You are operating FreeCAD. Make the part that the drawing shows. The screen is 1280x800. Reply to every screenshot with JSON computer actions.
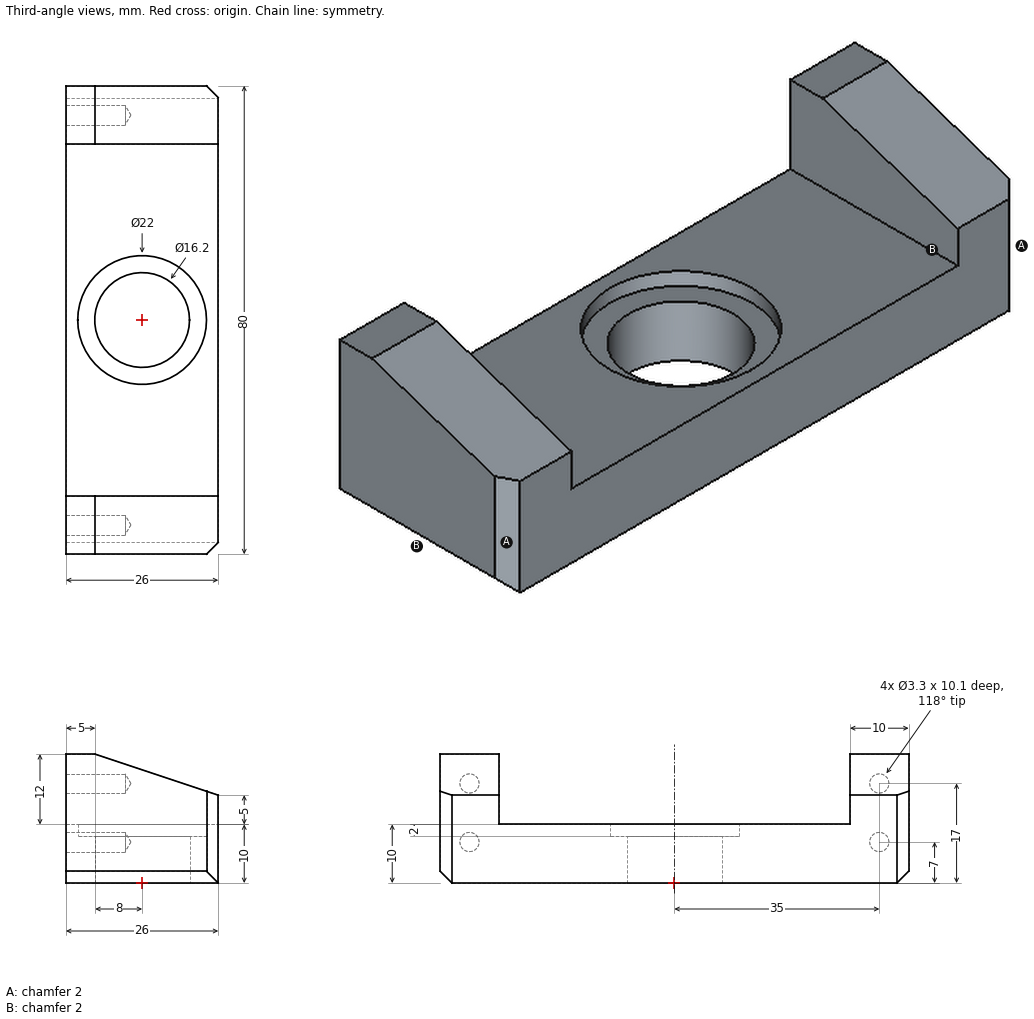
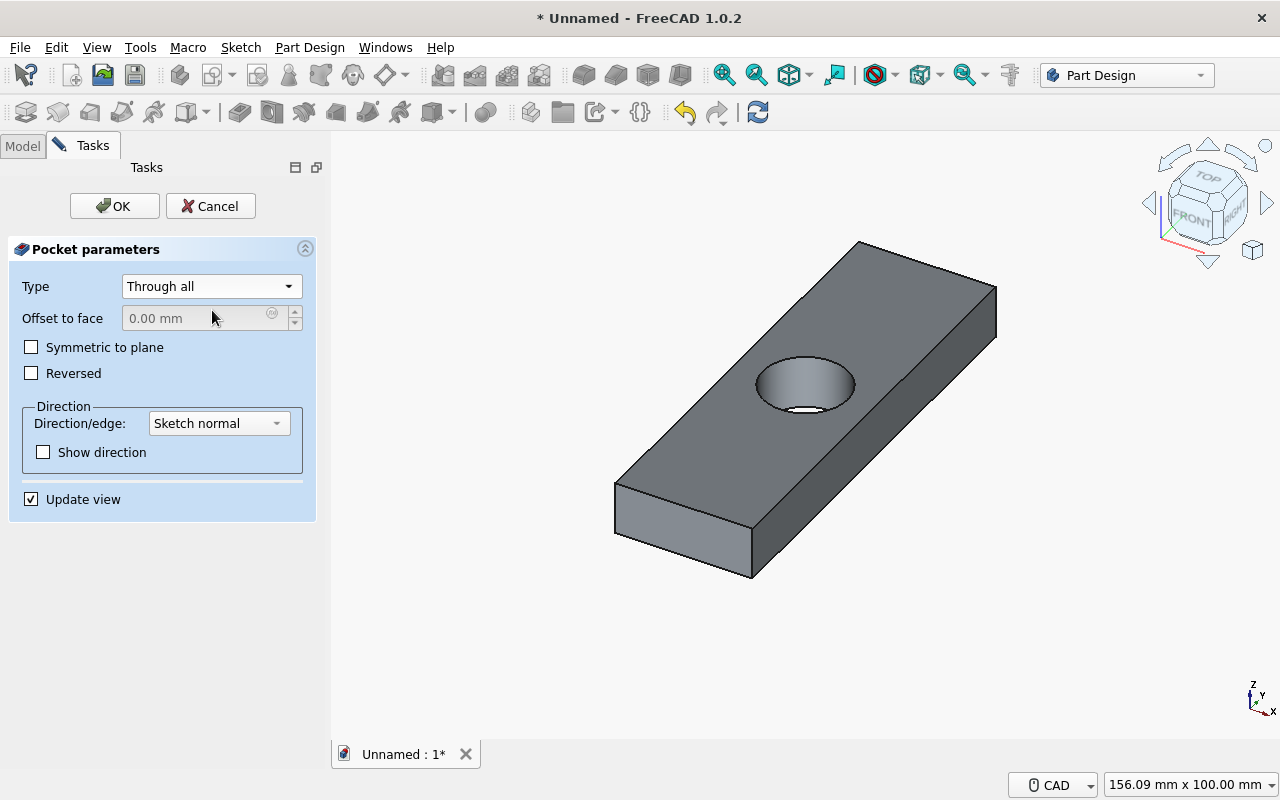
{"action": "left_click", "coordinate": [115, 206]}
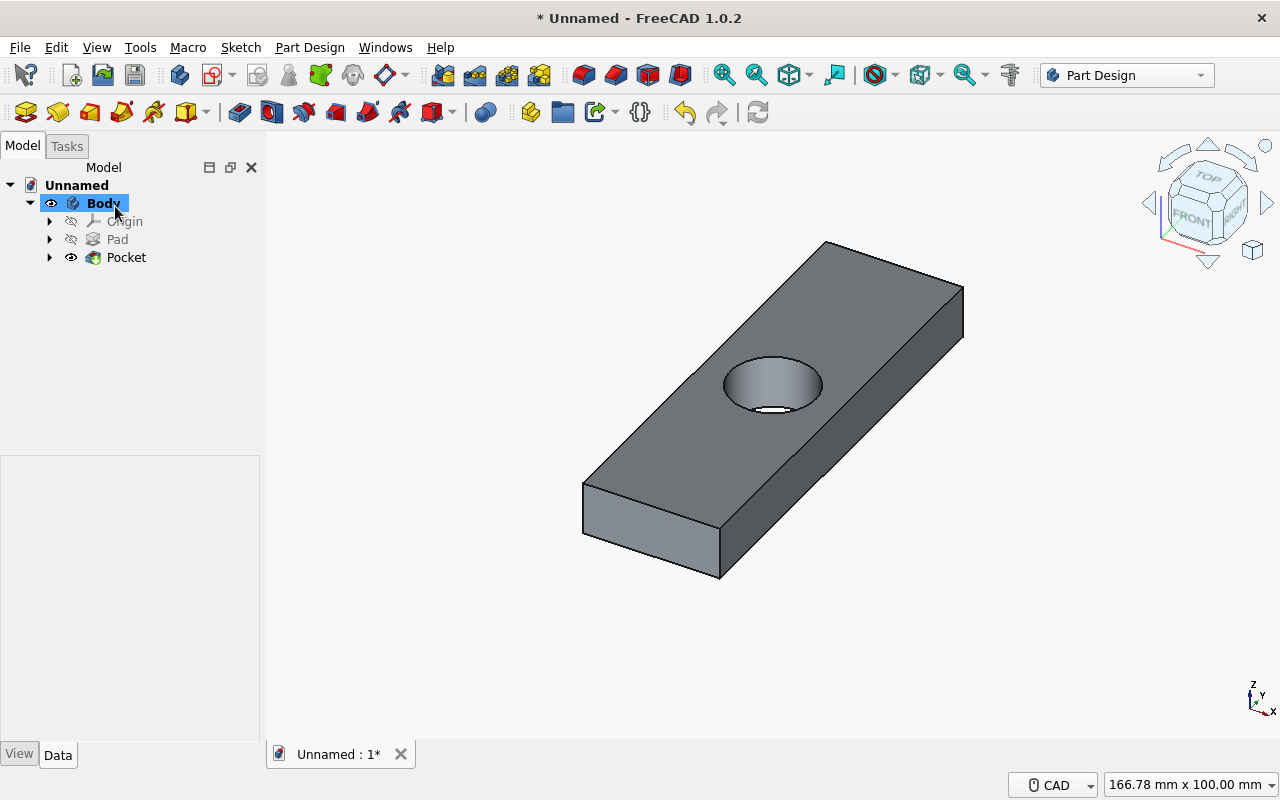
{"action": "key", "text": "4"}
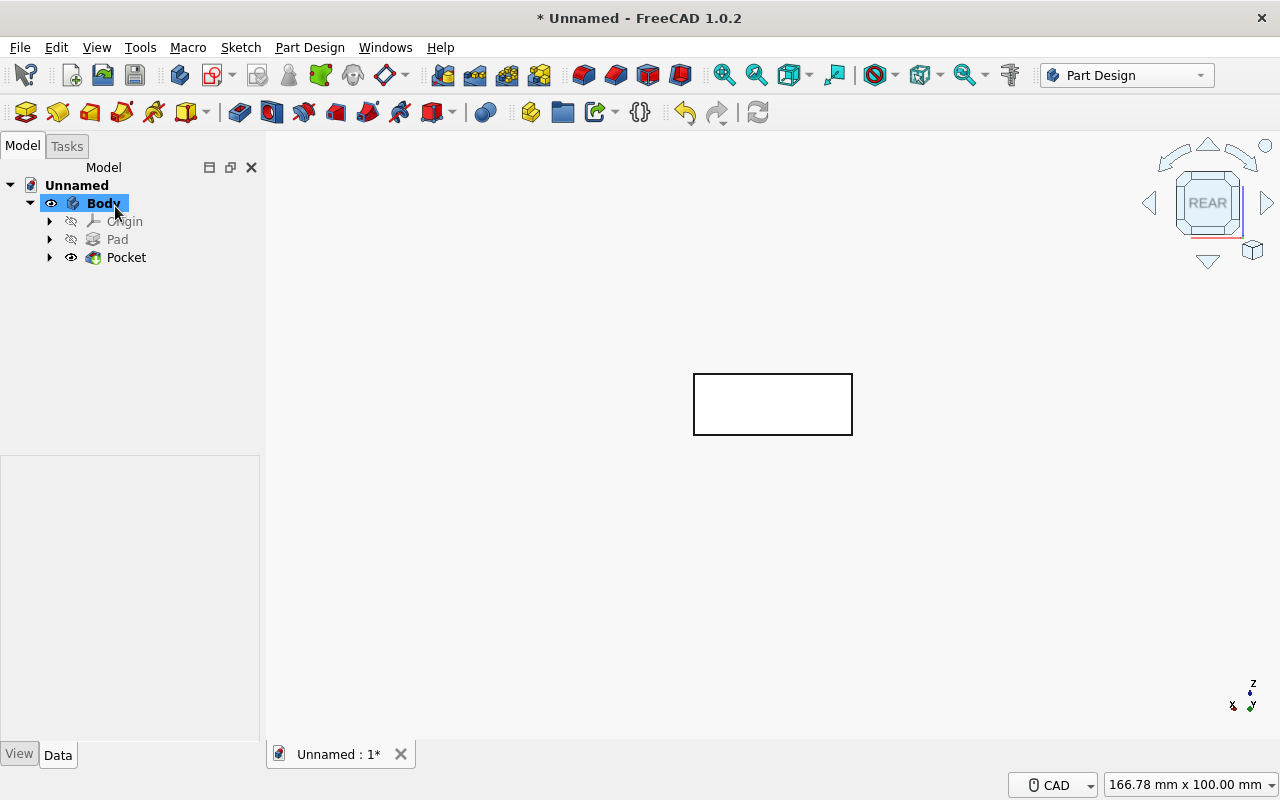
{"action": "left_click", "coordinate": [726, 76]}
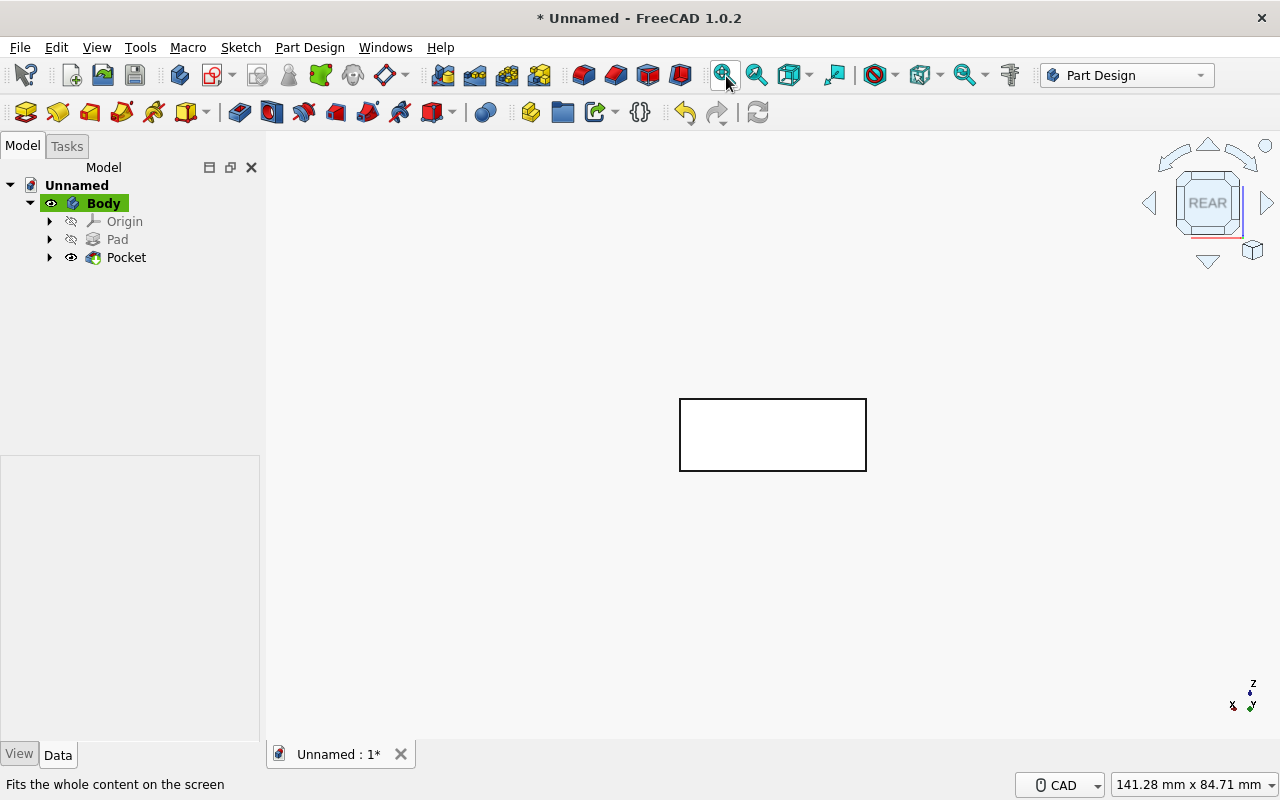
{"action": "left_click", "coordinate": [720, 434]}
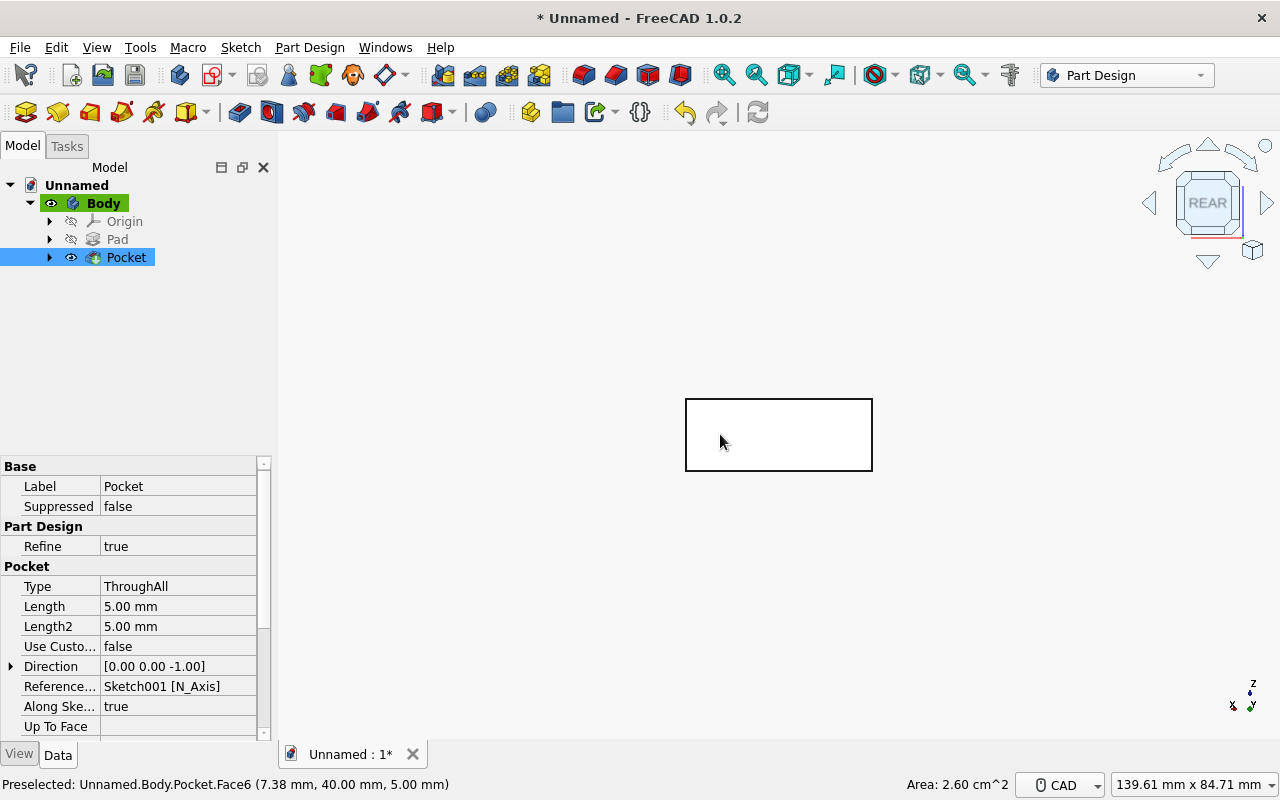
{"action": "left_click", "coordinate": [212, 76]}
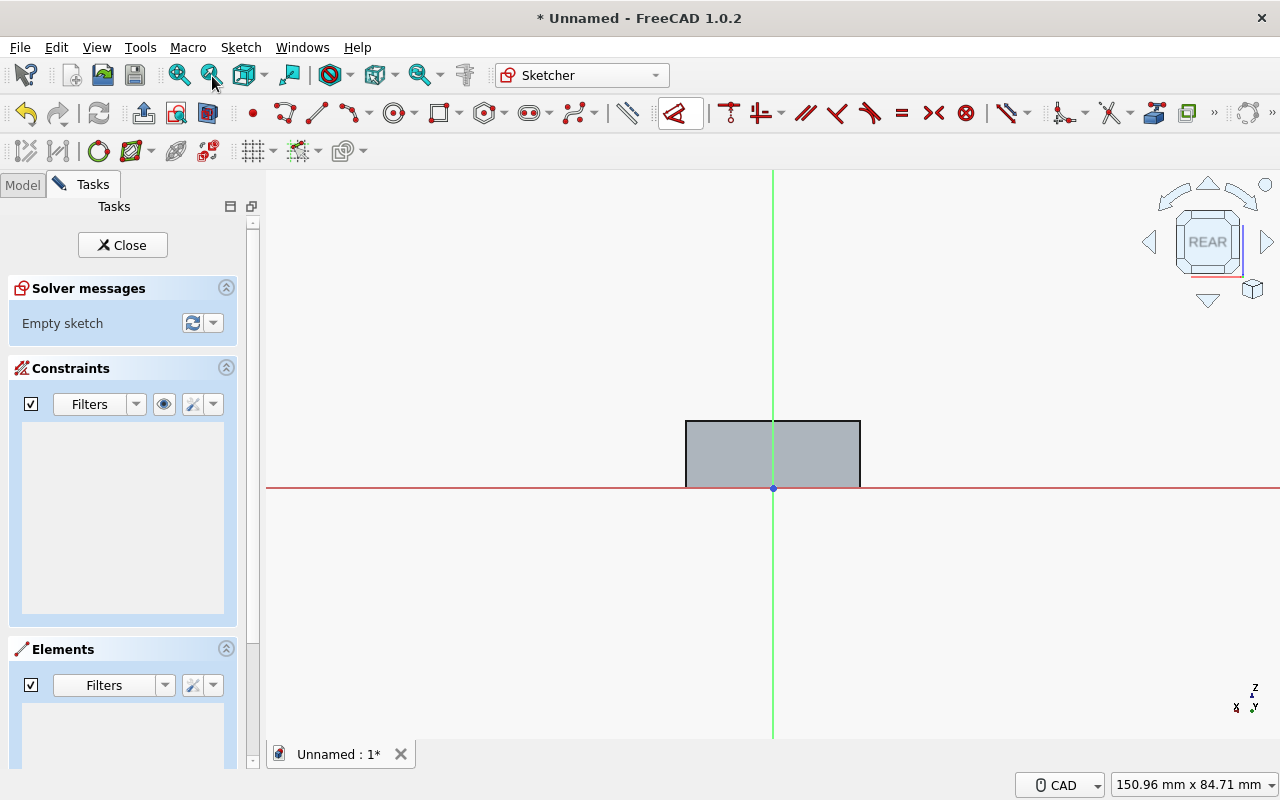
{"action": "scroll", "coordinate": [829, 381], "scroll_direction": "up", "scroll_amount": 4}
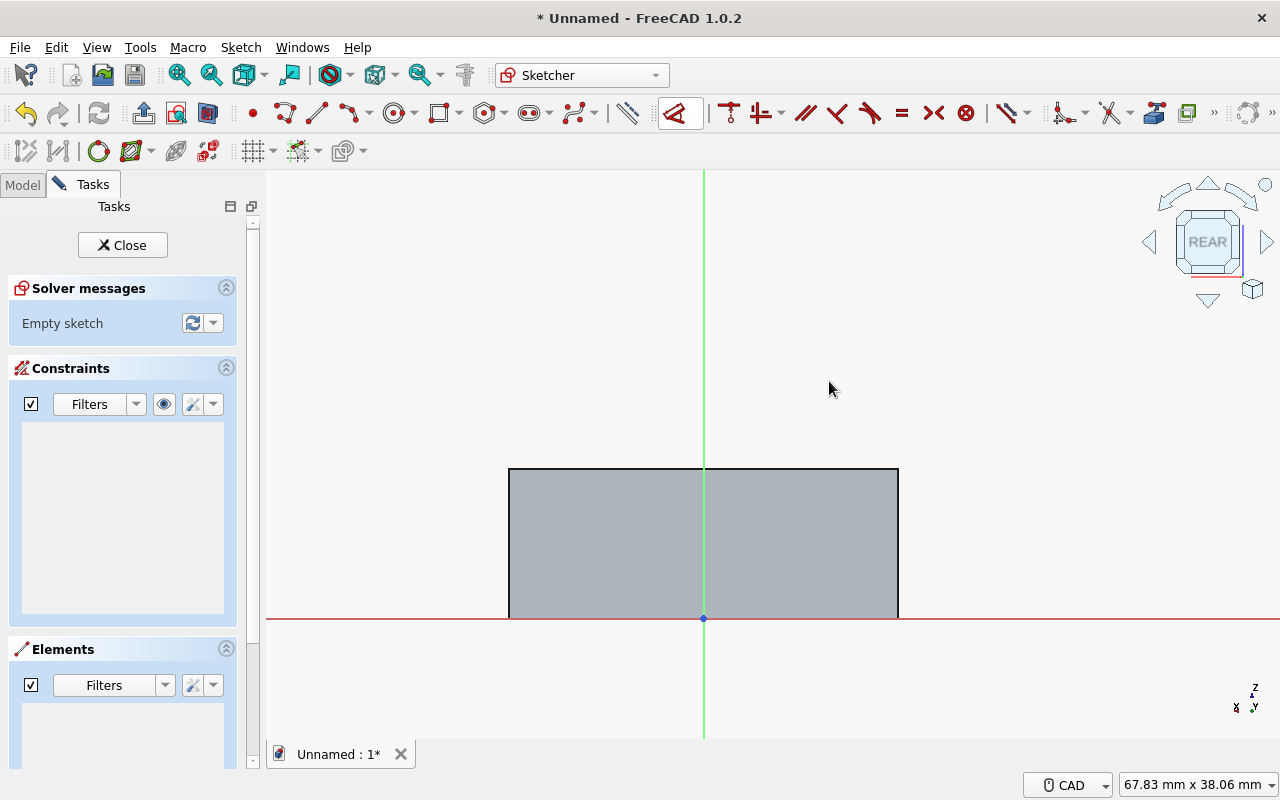
{"action": "left_click", "coordinate": [286, 114]}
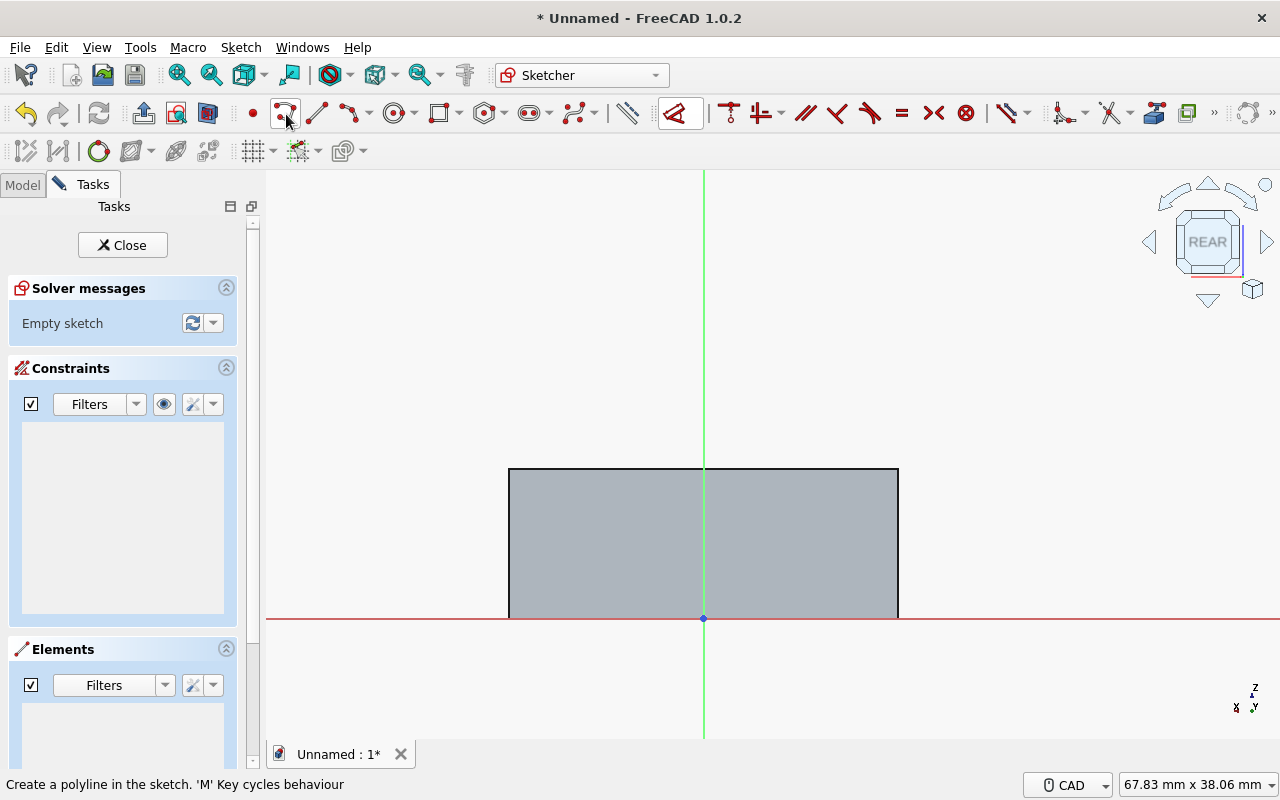
{"action": "left_click", "coordinate": [509, 469]}
{"action": "left_click", "coordinate": [898, 469]}
{"action": "left_click", "coordinate": [898, 290]}
{"action": "left_click", "coordinate": [823, 290]}
{"action": "left_click", "coordinate": [509, 395]}
{"action": "left_click", "coordinate": [509, 470]}
{"action": "key", "text": "Escape"}
{"action": "key", "text": "Escape"}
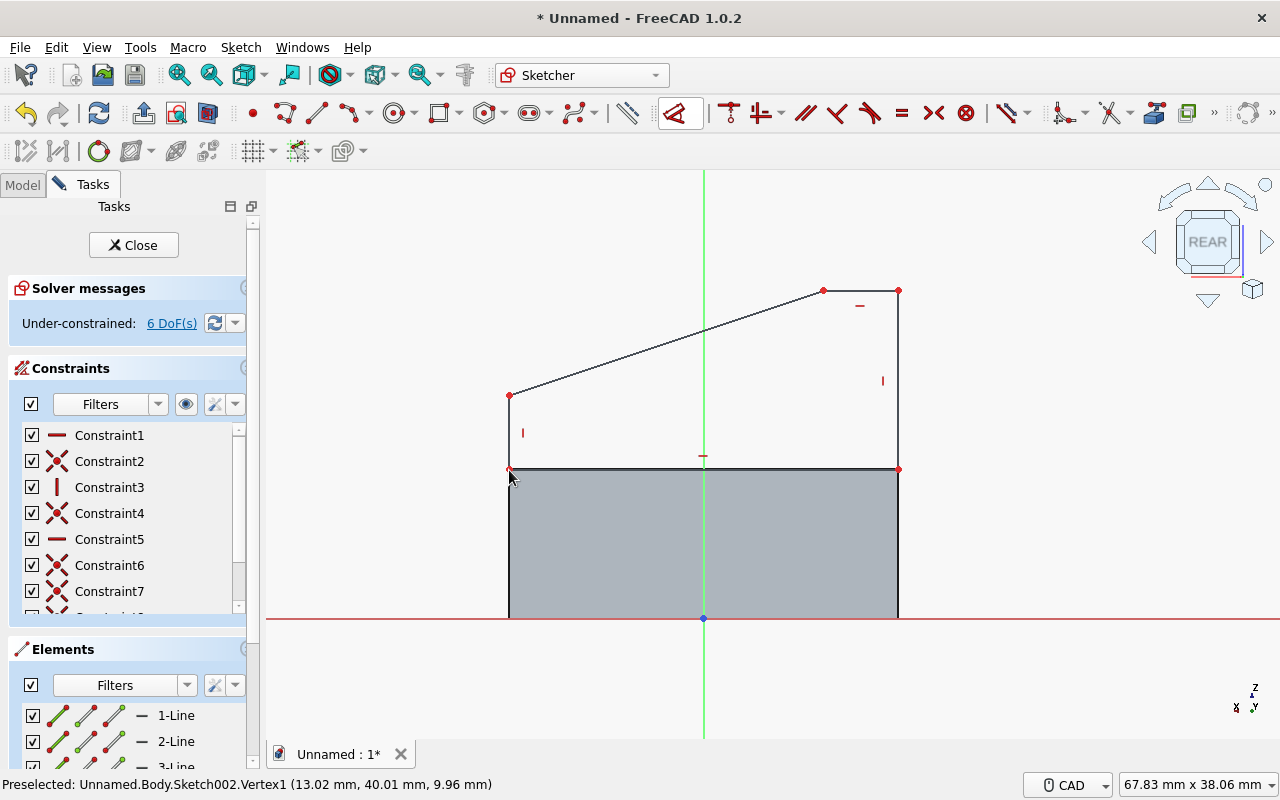
{"action": "left_click", "coordinate": [875, 291]}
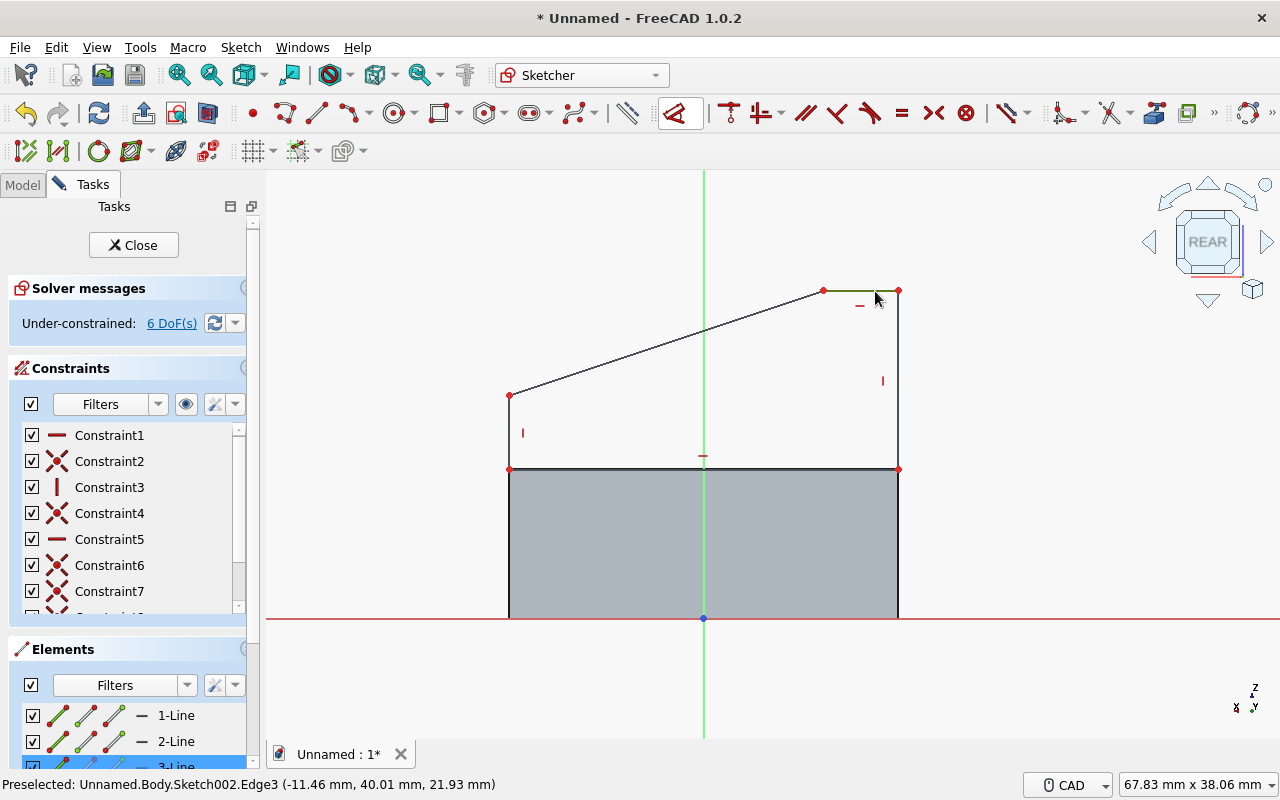
{"action": "key", "text": "l"}